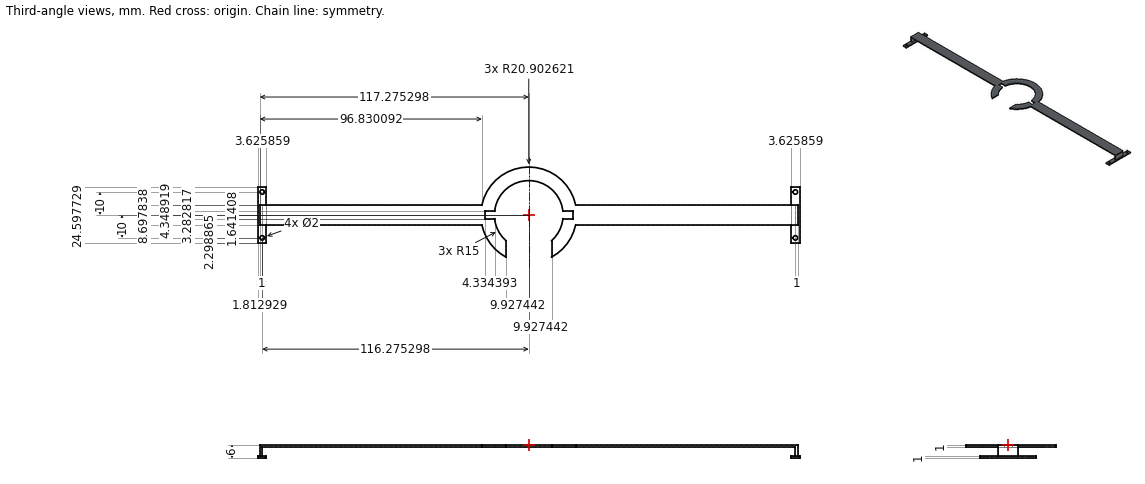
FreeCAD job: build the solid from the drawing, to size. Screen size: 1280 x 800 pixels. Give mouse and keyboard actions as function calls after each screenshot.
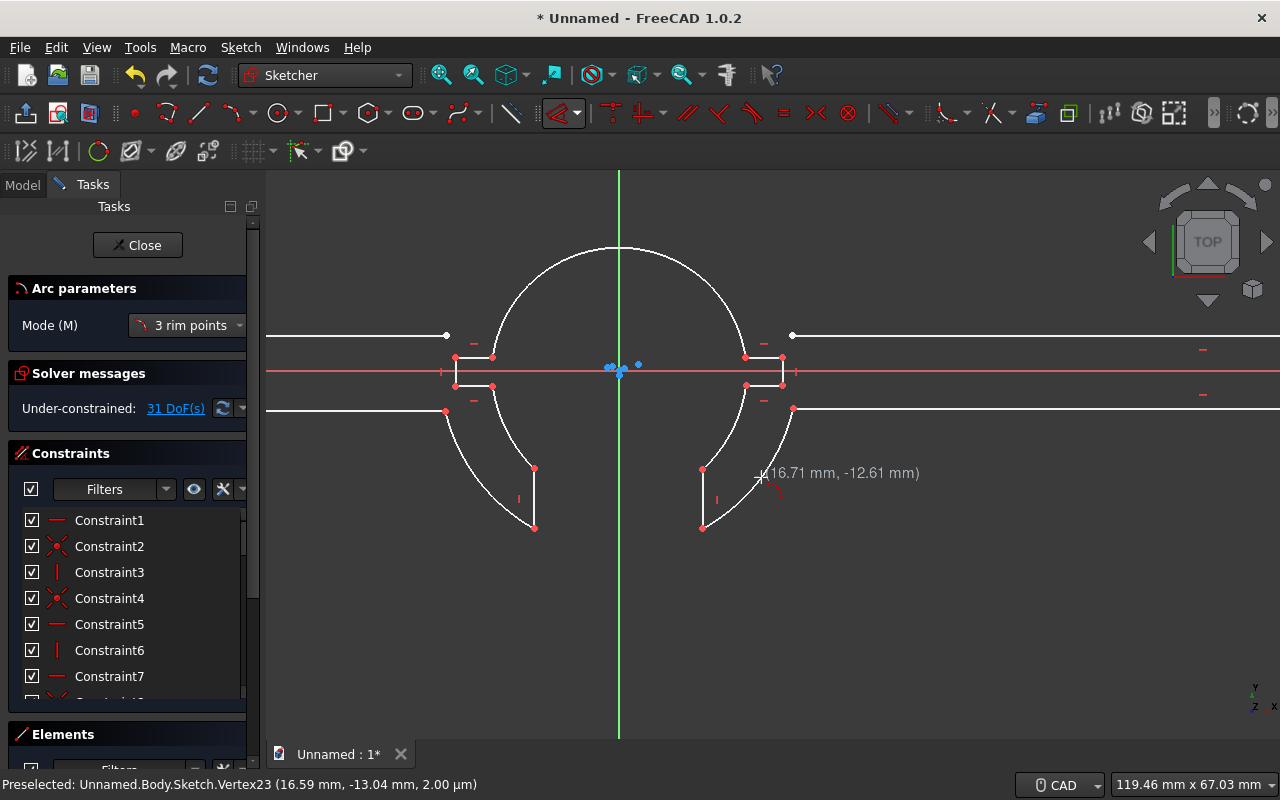
click(792, 336)
click(447, 336)
click(667, 200)
key(Escape)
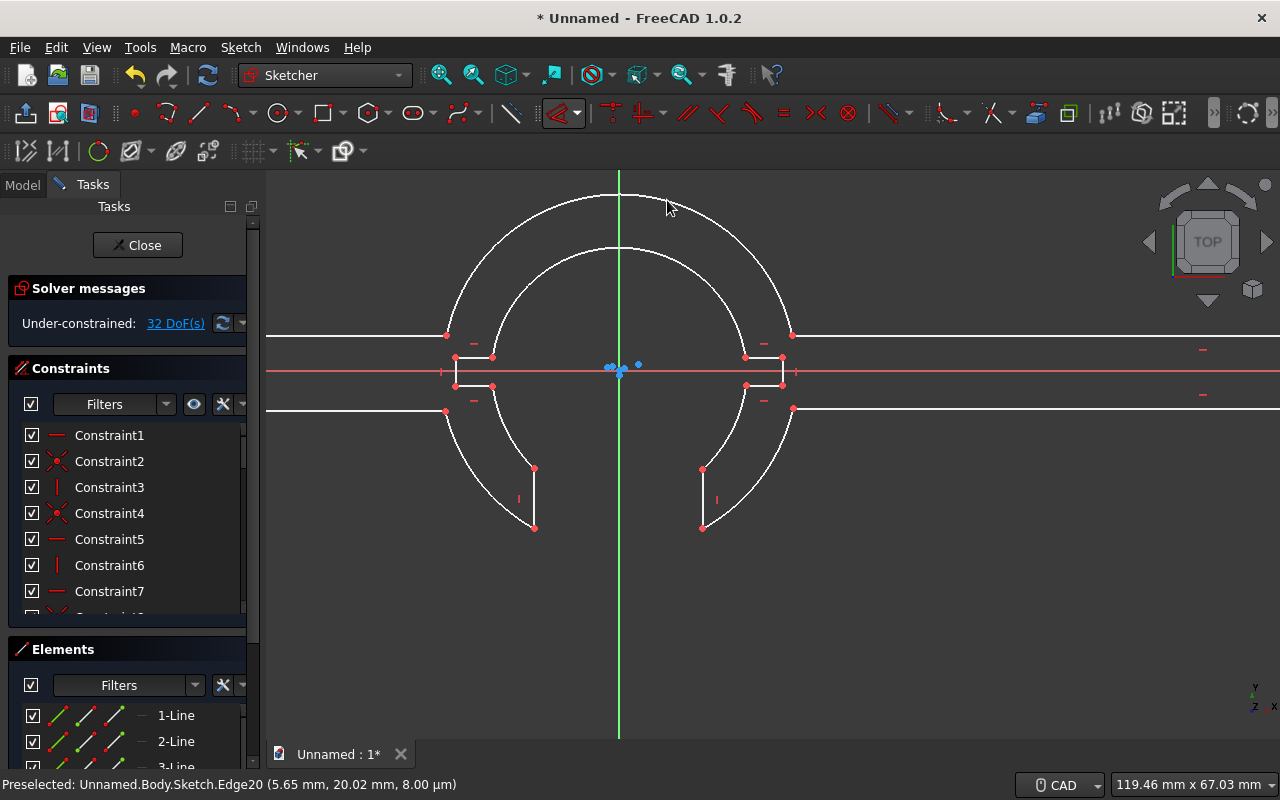
click(461, 454)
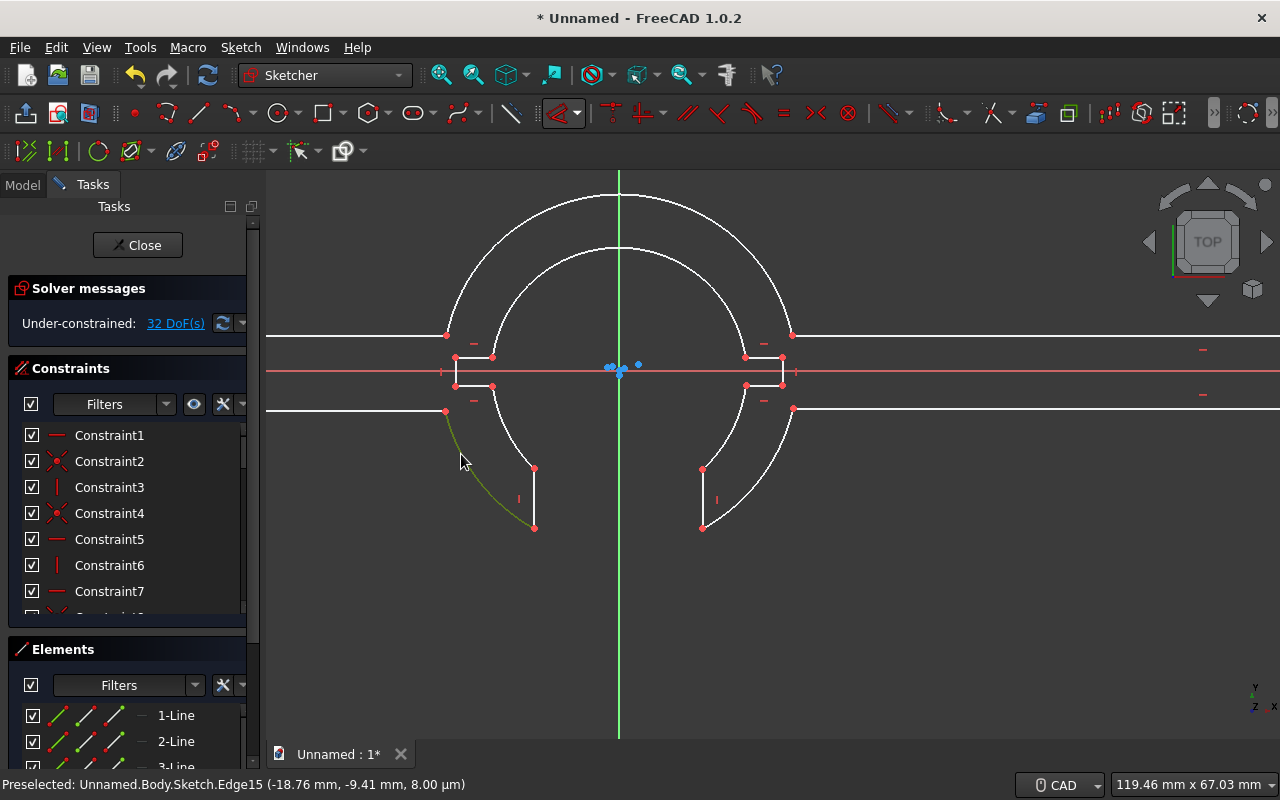
click(499, 413)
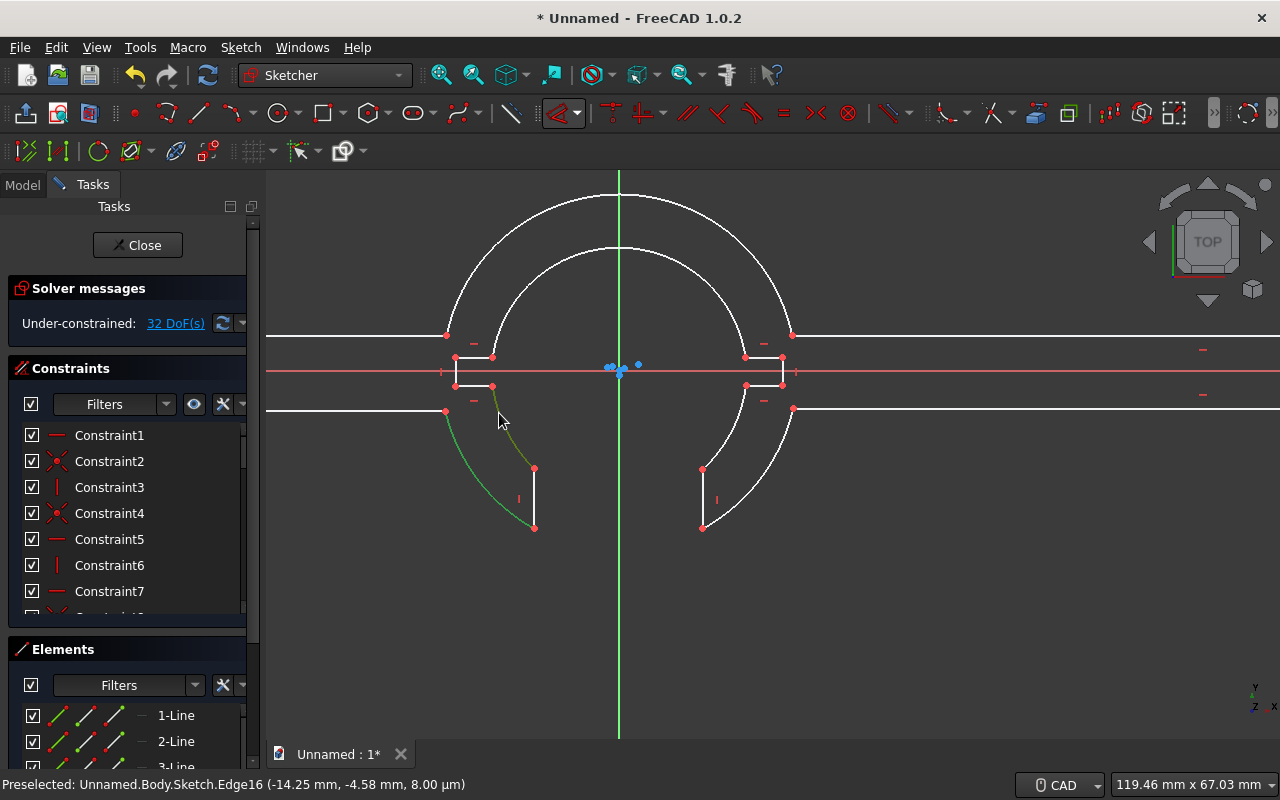
key(c)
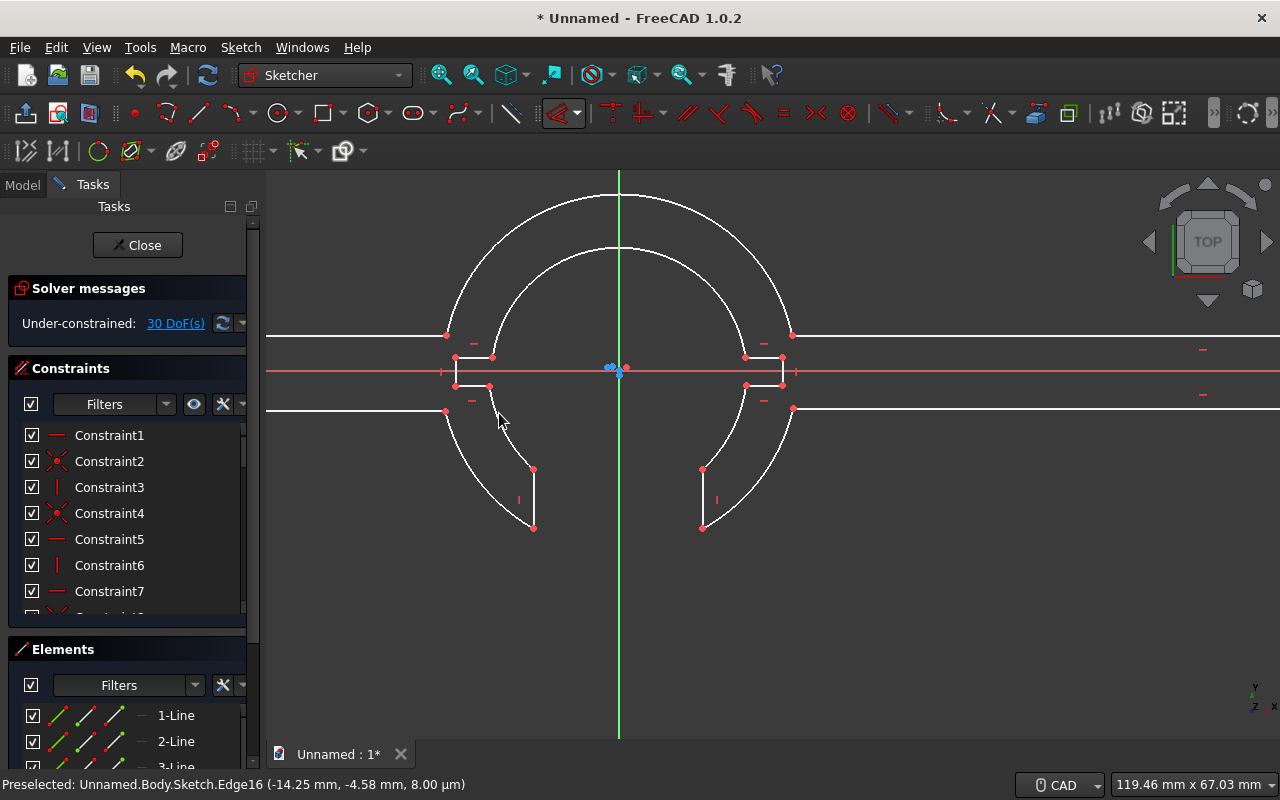
click(461, 453)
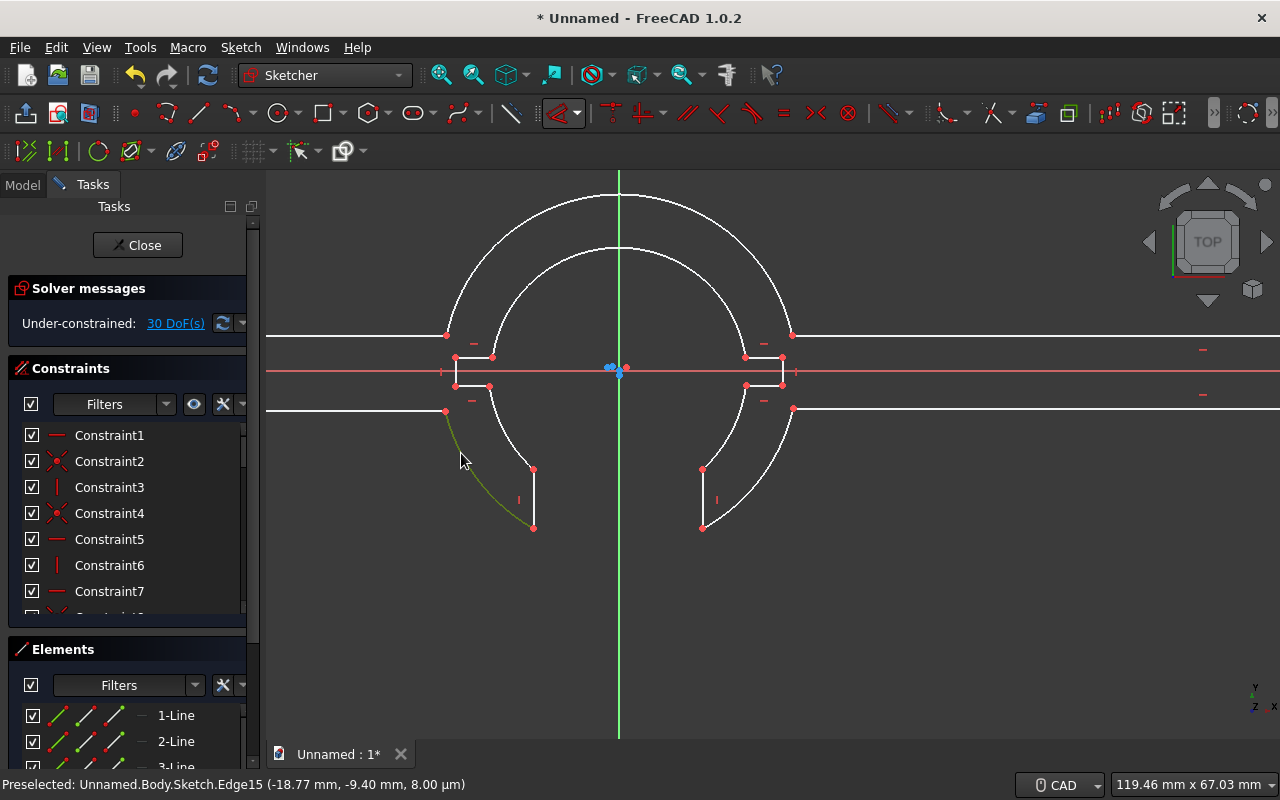
click(688, 268)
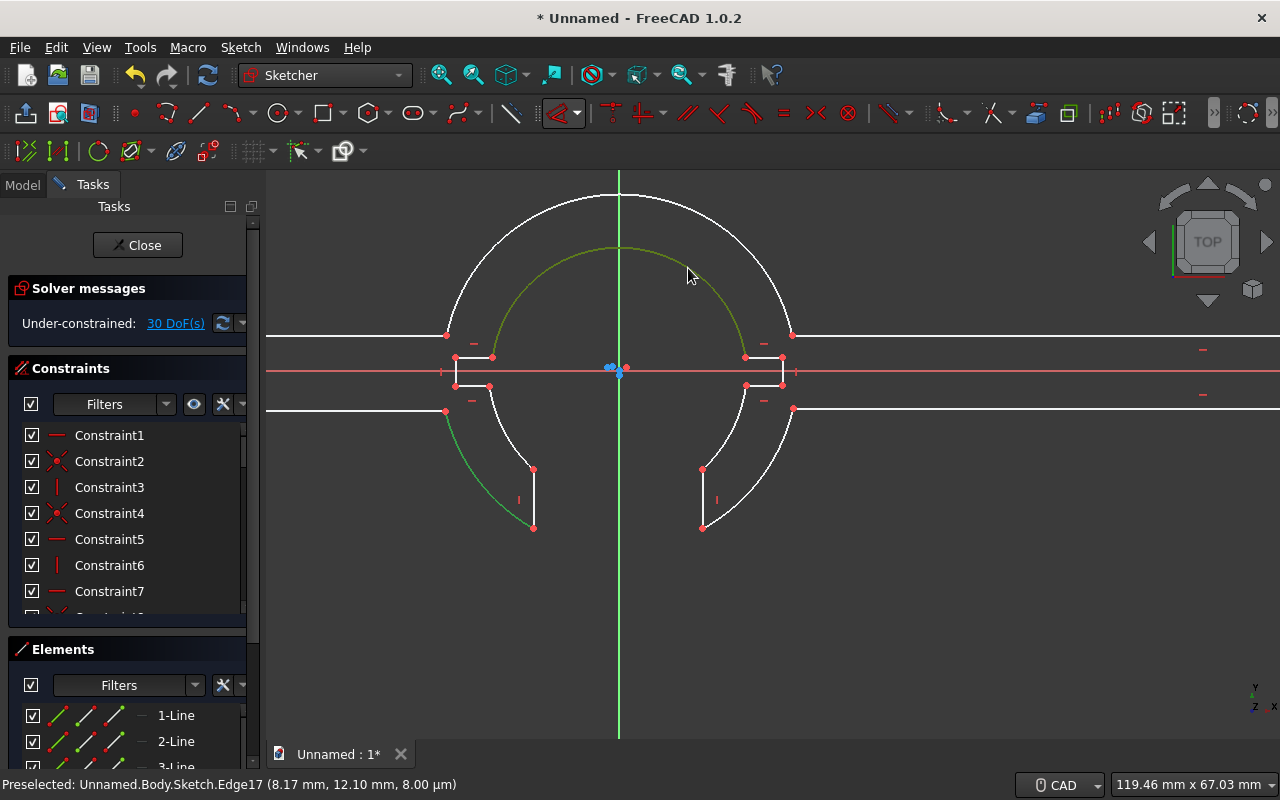
click(612, 114)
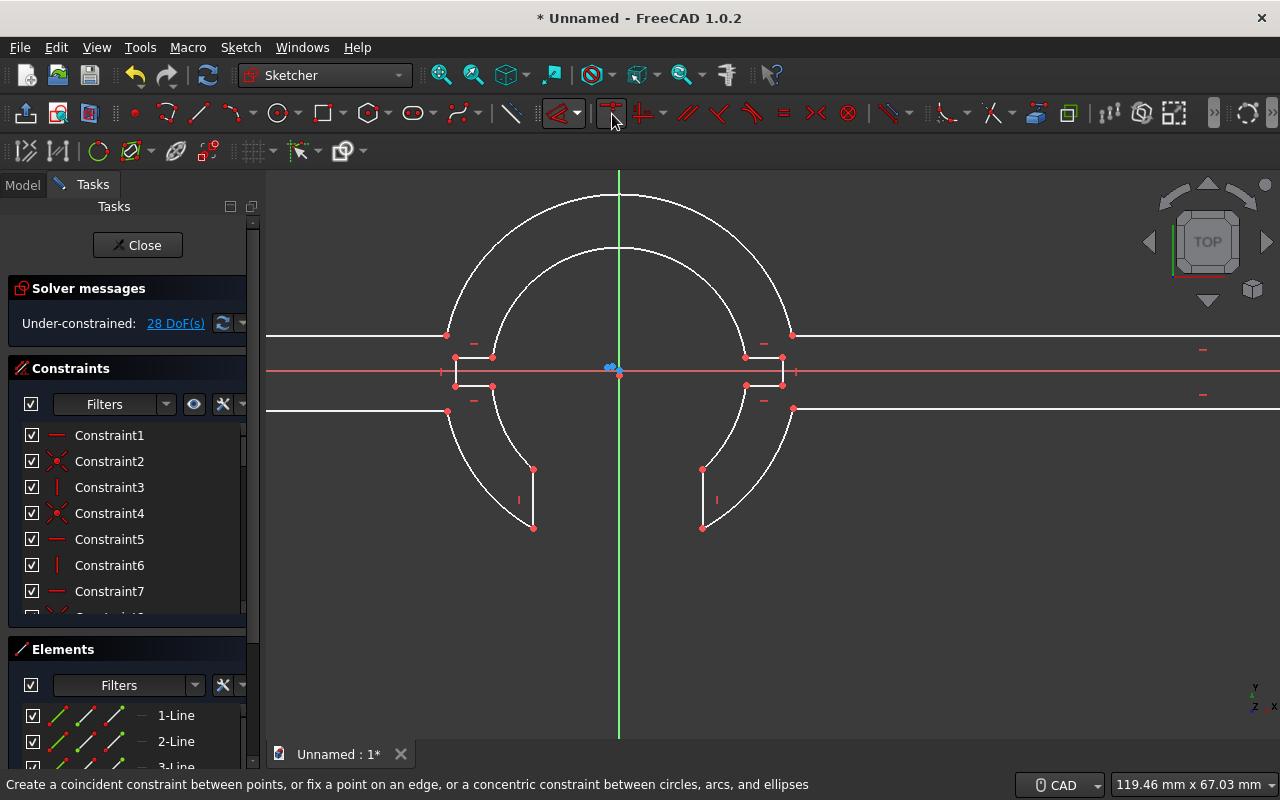
click(462, 454)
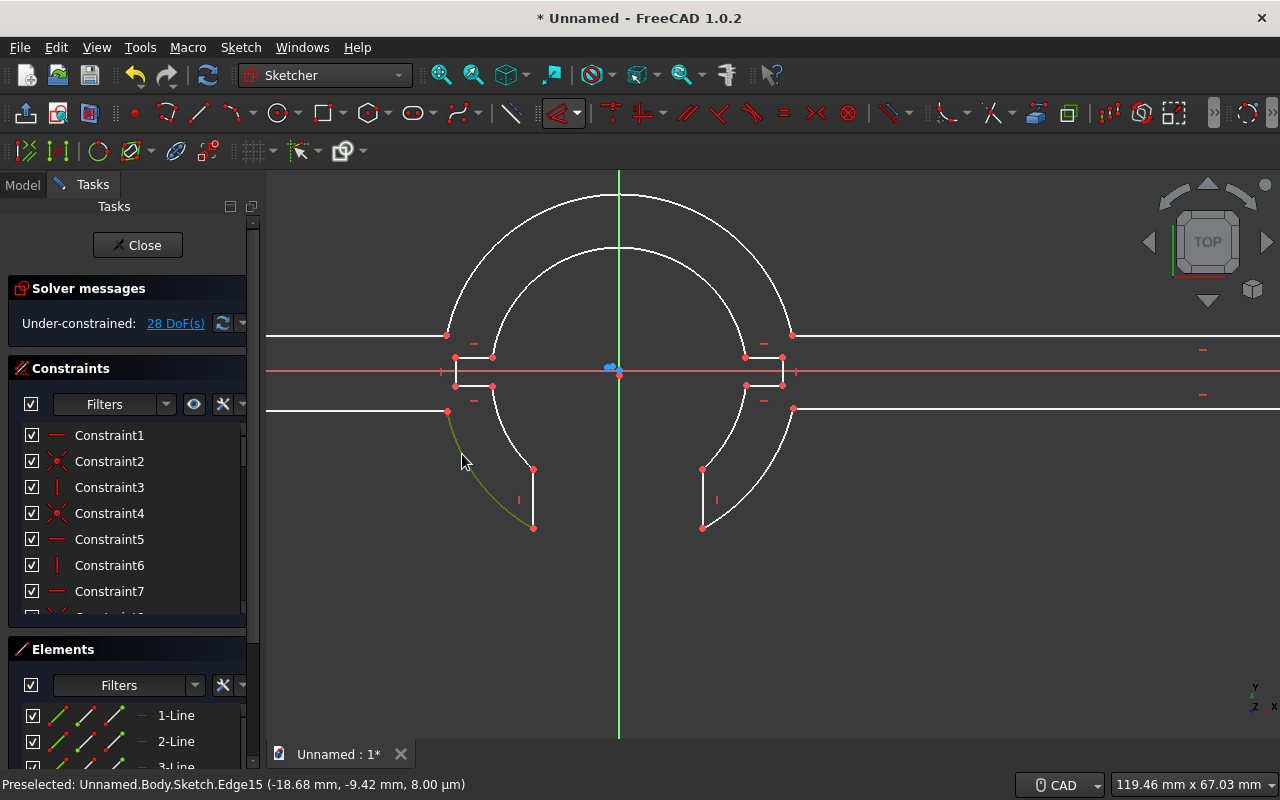
click(722, 448)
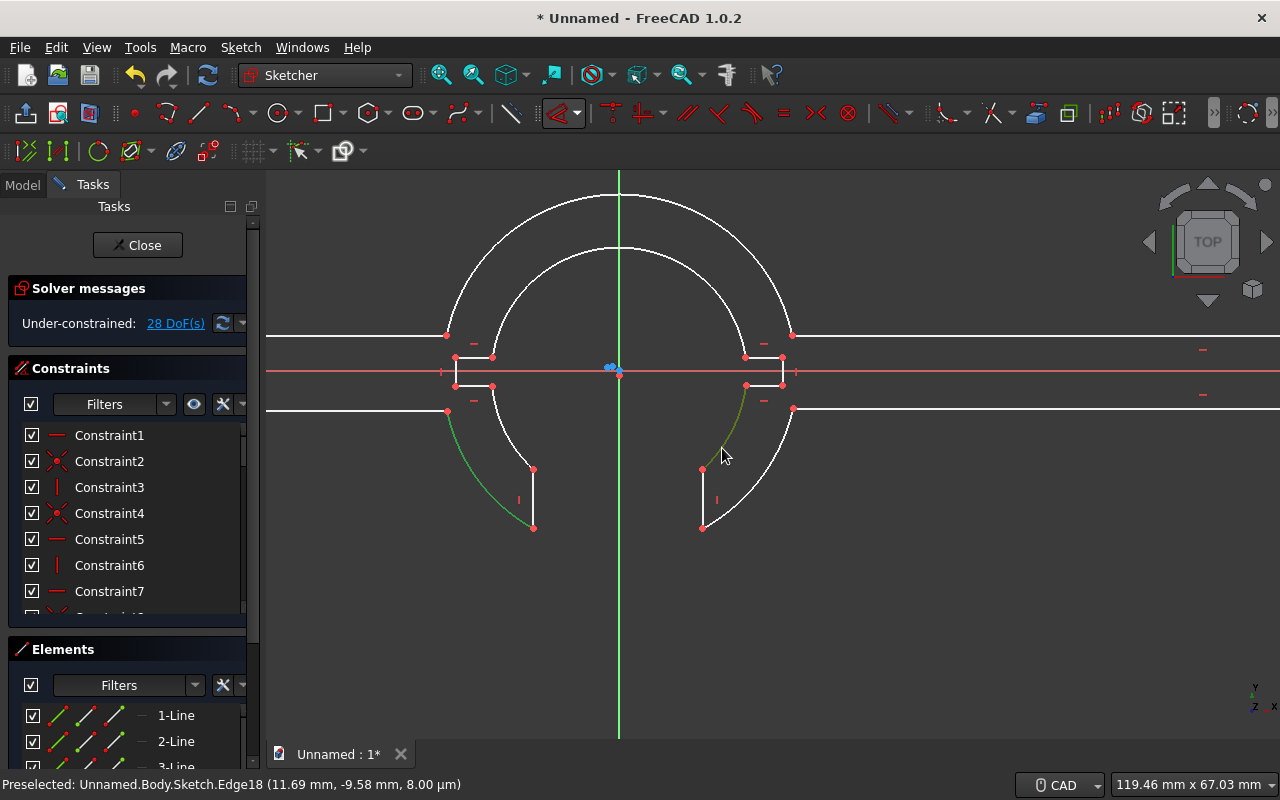
click(612, 114)